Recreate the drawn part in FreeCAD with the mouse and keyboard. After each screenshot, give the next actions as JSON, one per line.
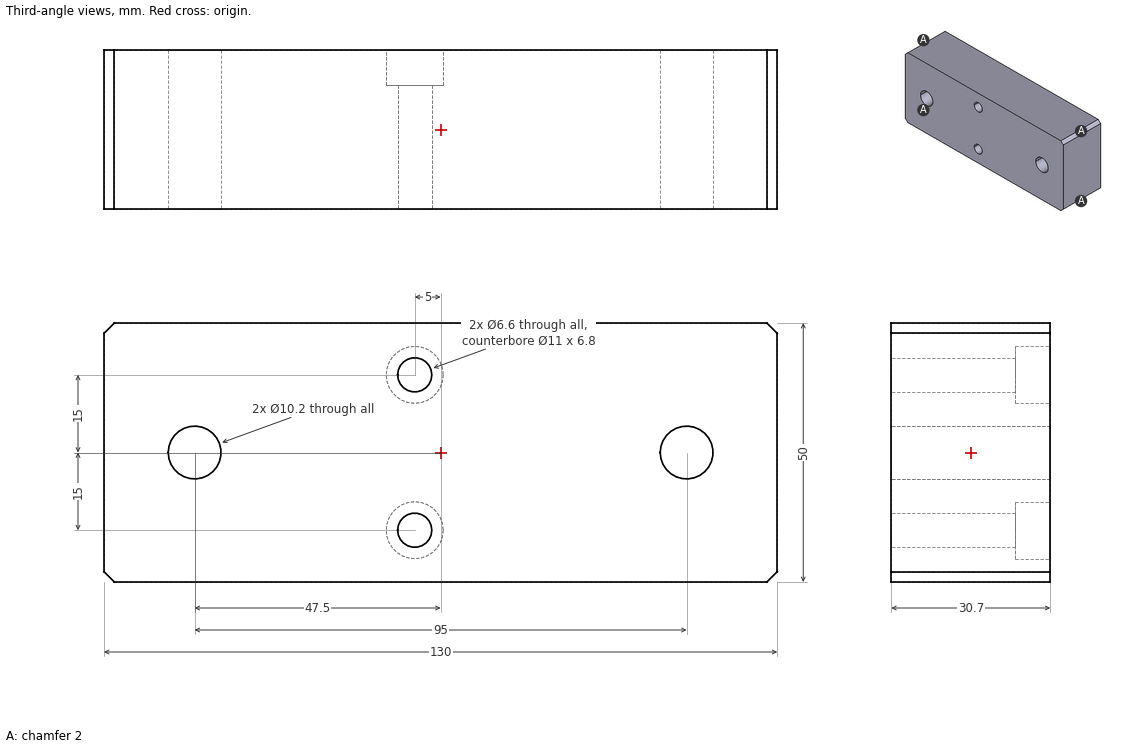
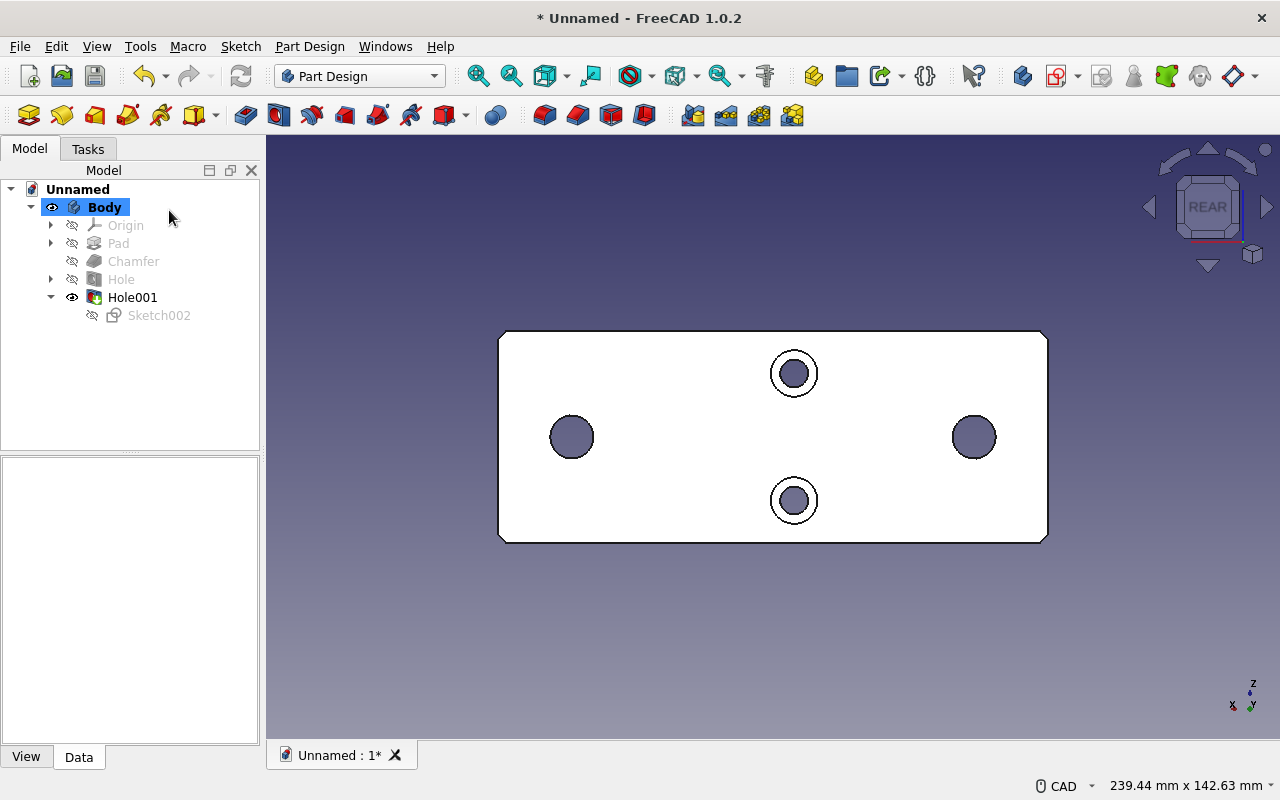
{"action": "key", "text": "0"}